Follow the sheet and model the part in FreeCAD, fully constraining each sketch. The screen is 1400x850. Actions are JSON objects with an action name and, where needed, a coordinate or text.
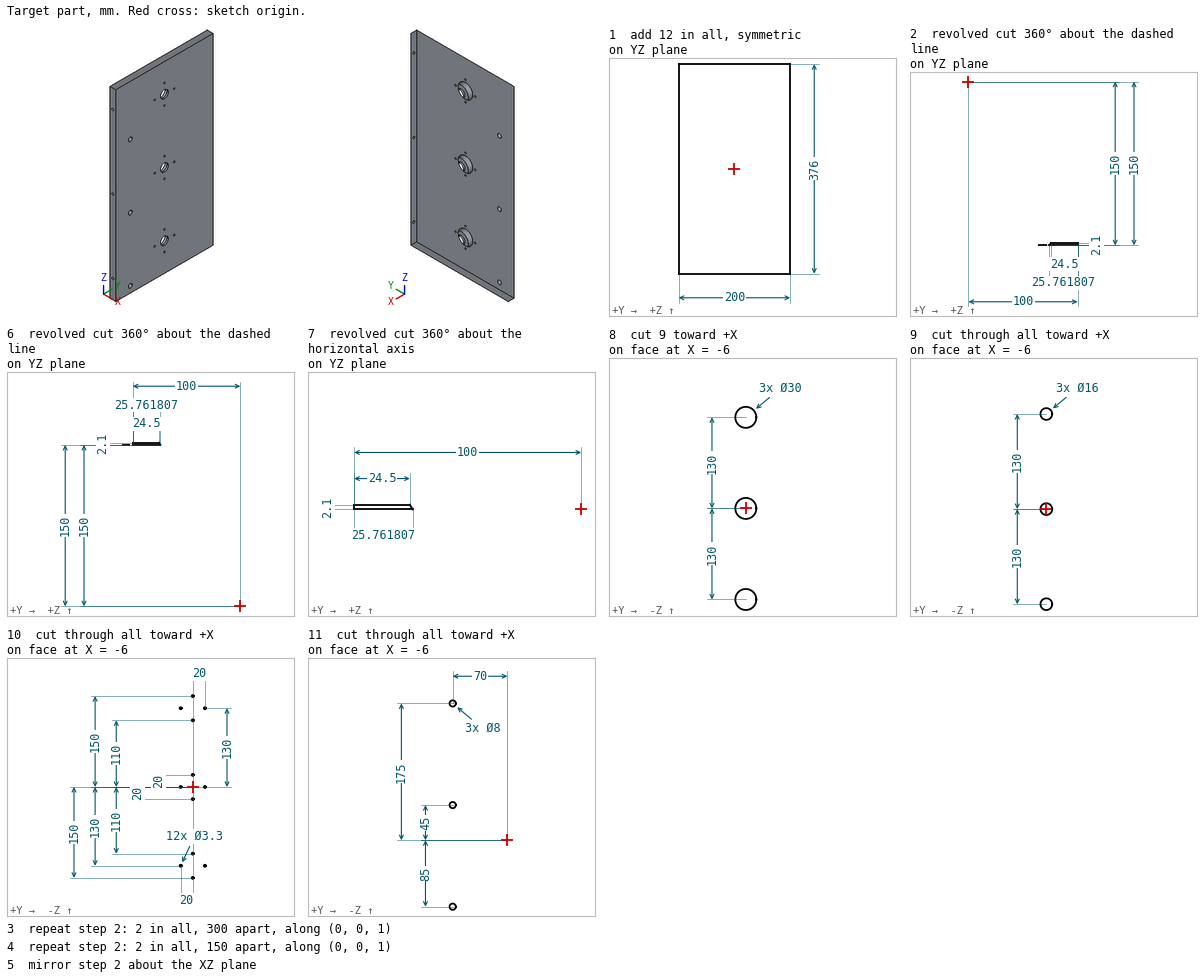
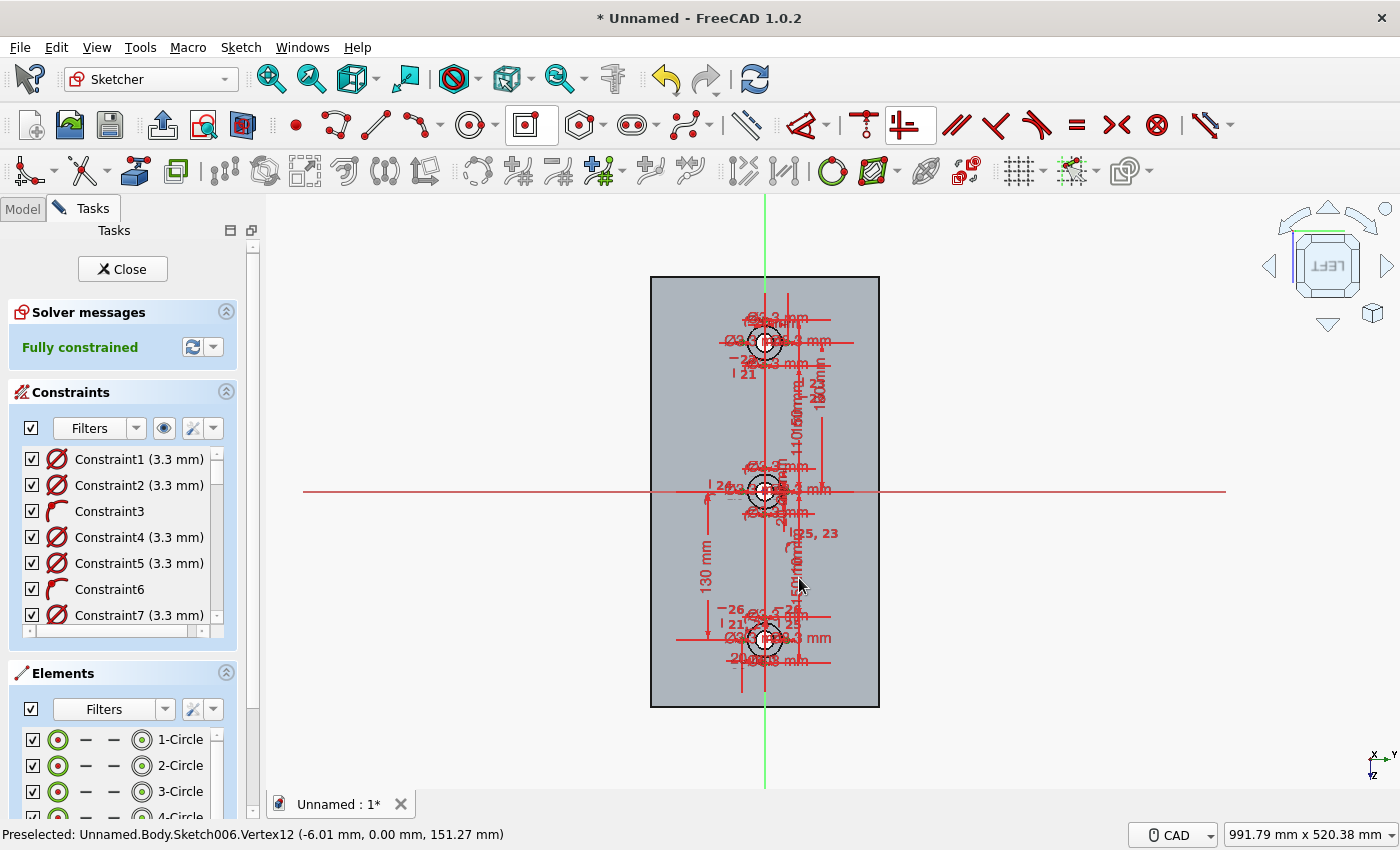
{"action": "left_click", "coordinate": [123, 269]}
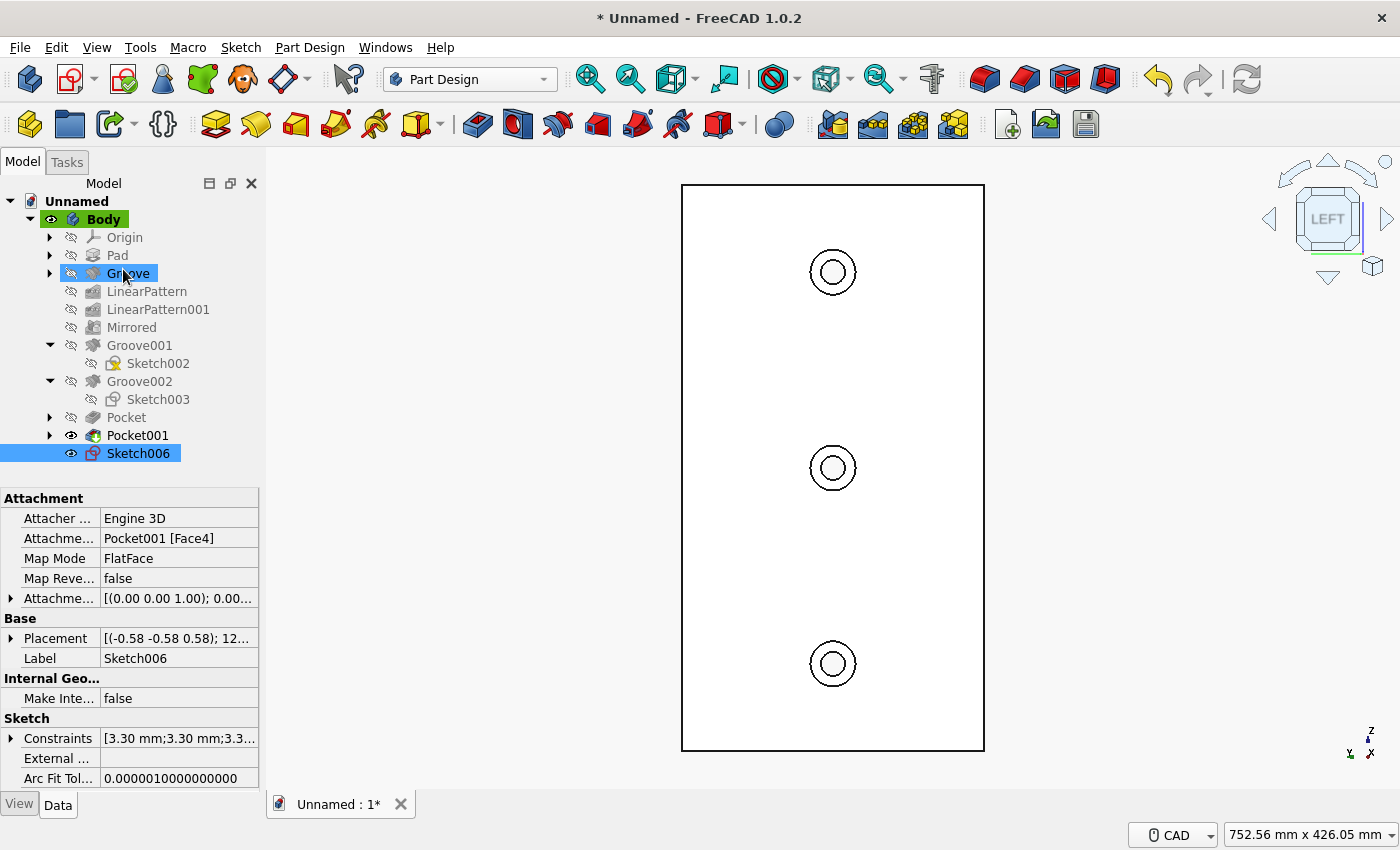
{"action": "left_click", "coordinate": [478, 124]}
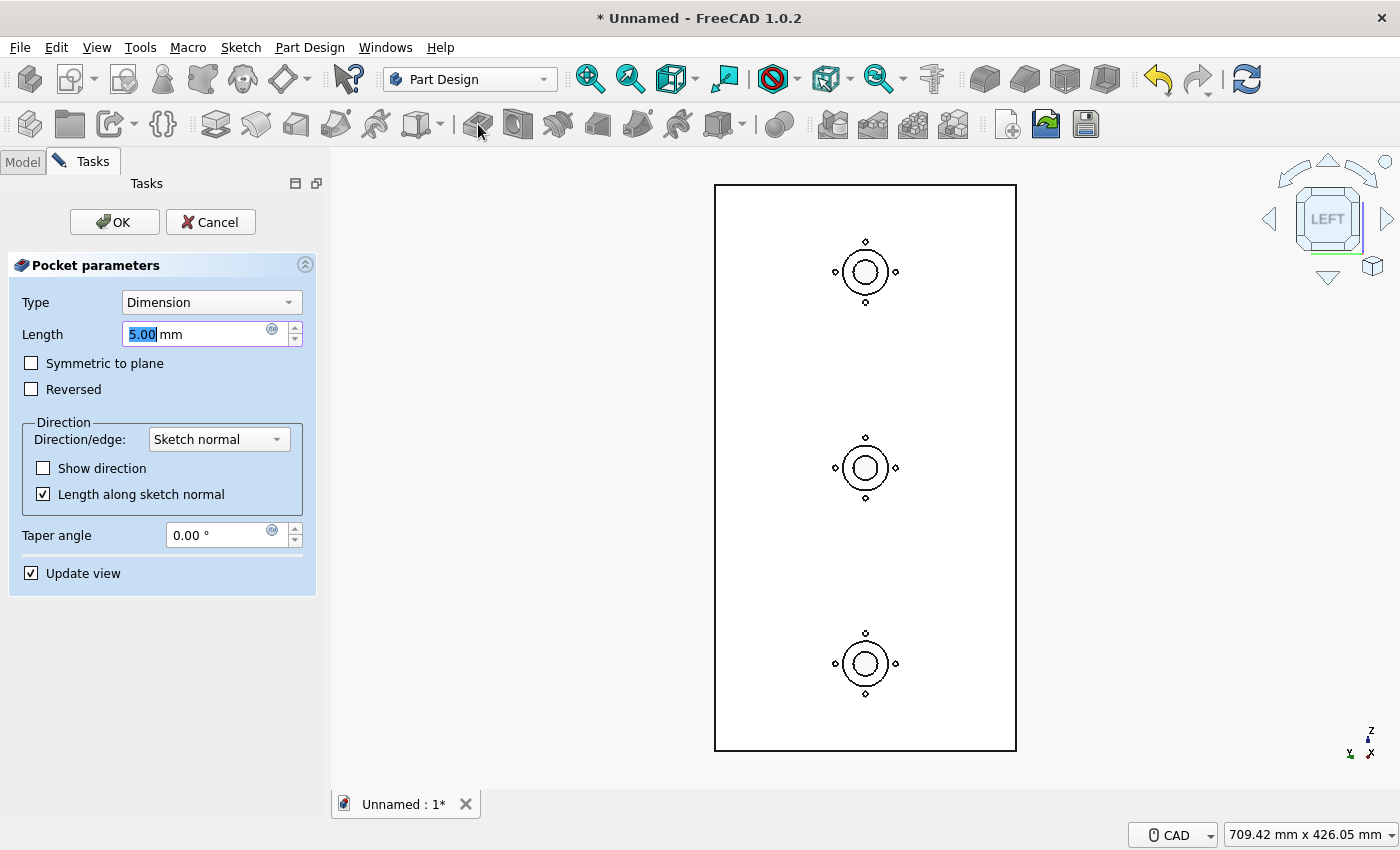
{"action": "left_click", "coordinate": [212, 302]}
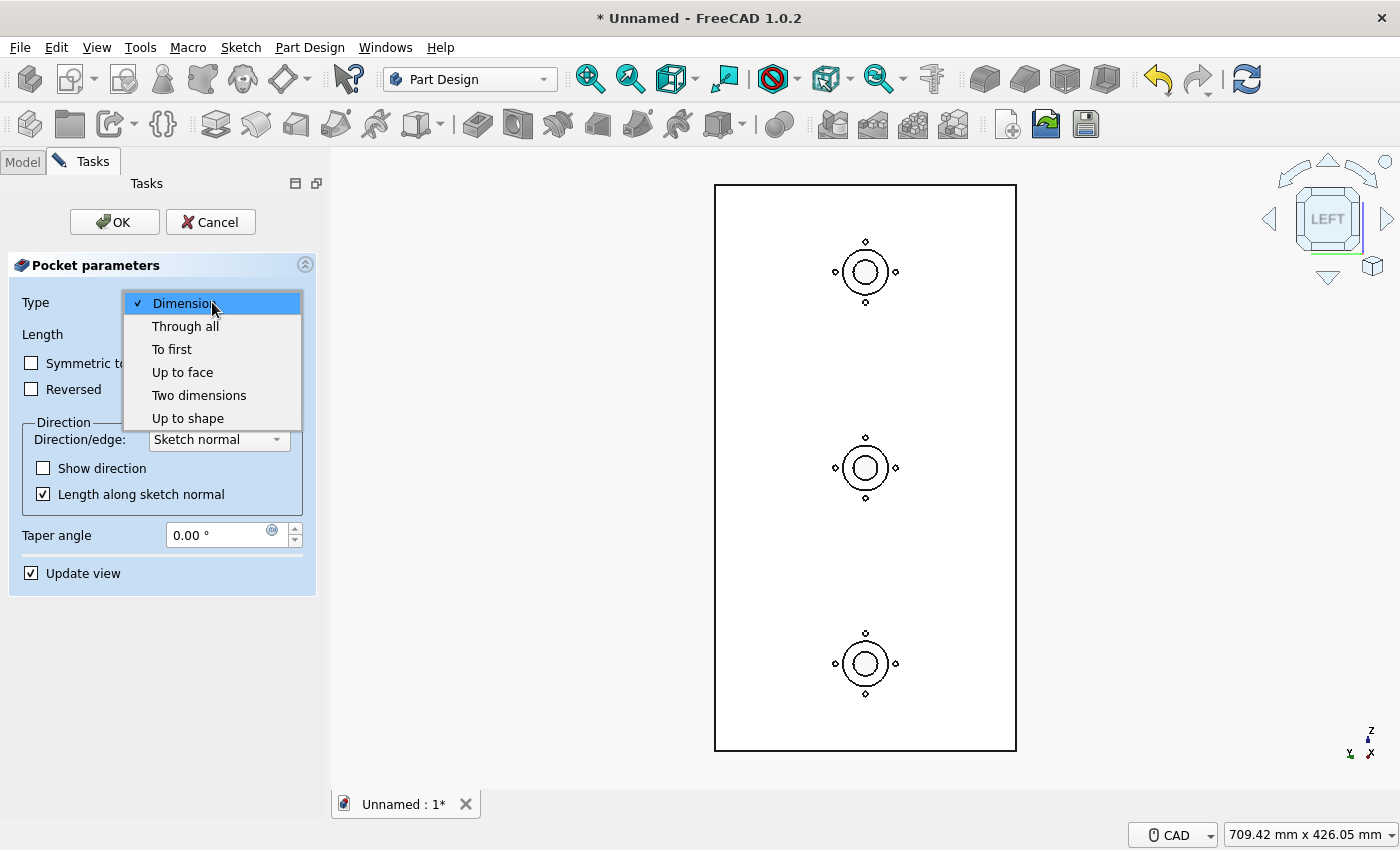
{"action": "left_click", "coordinate": [212, 326]}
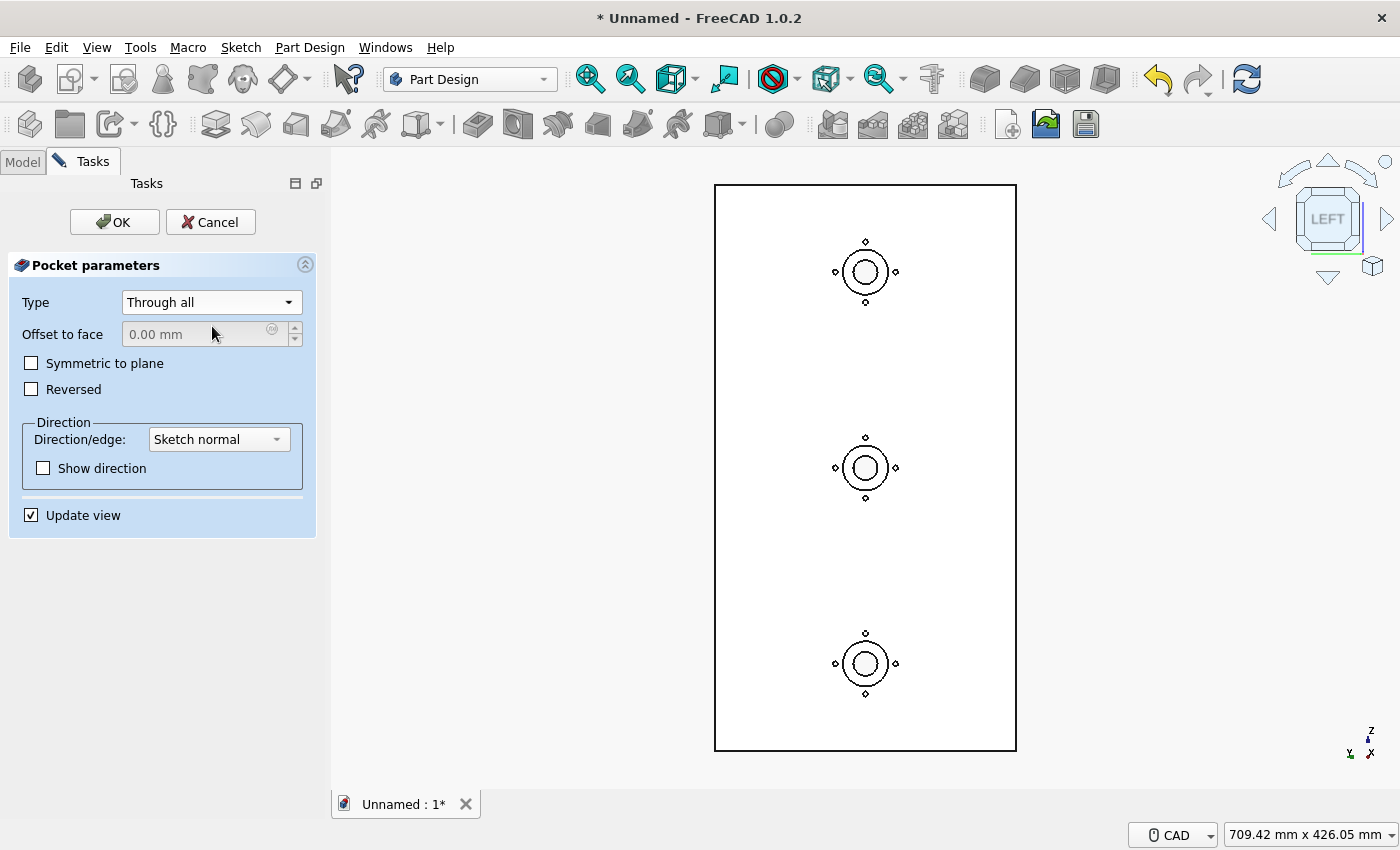
{"action": "left_click", "coordinate": [115, 222]}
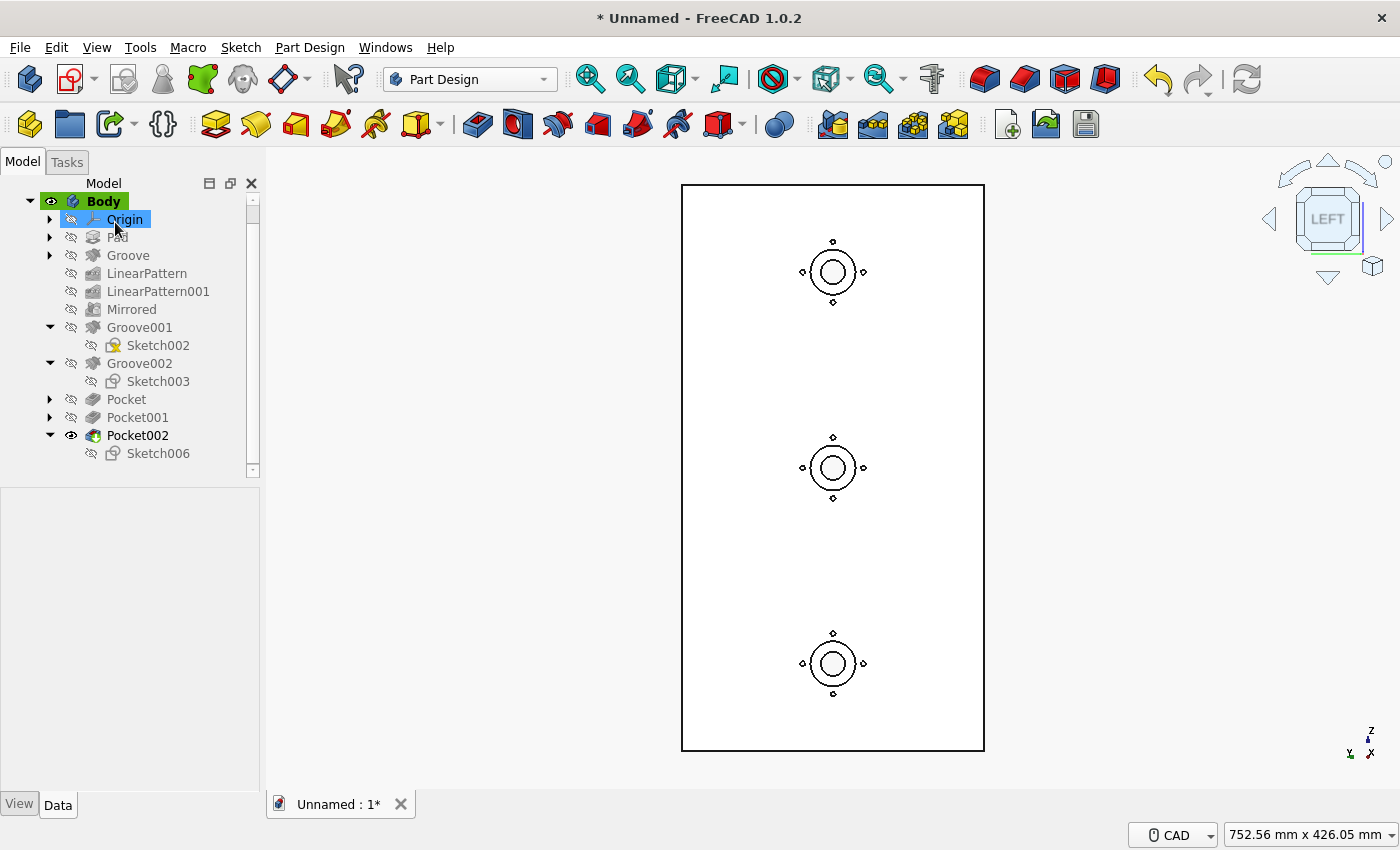
{"action": "left_click", "coordinate": [747, 548]}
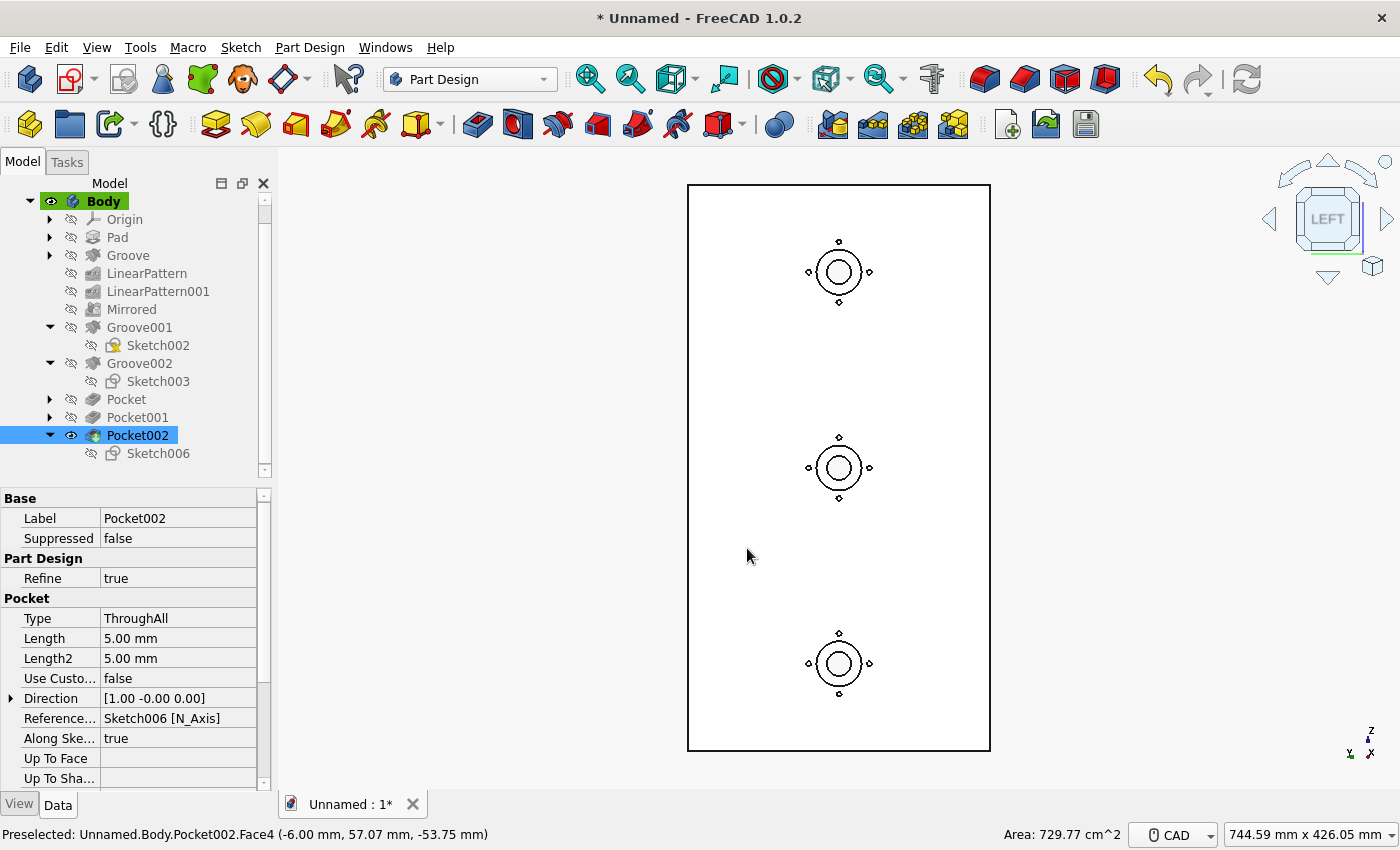
{"action": "left_click", "coordinate": [70, 80]}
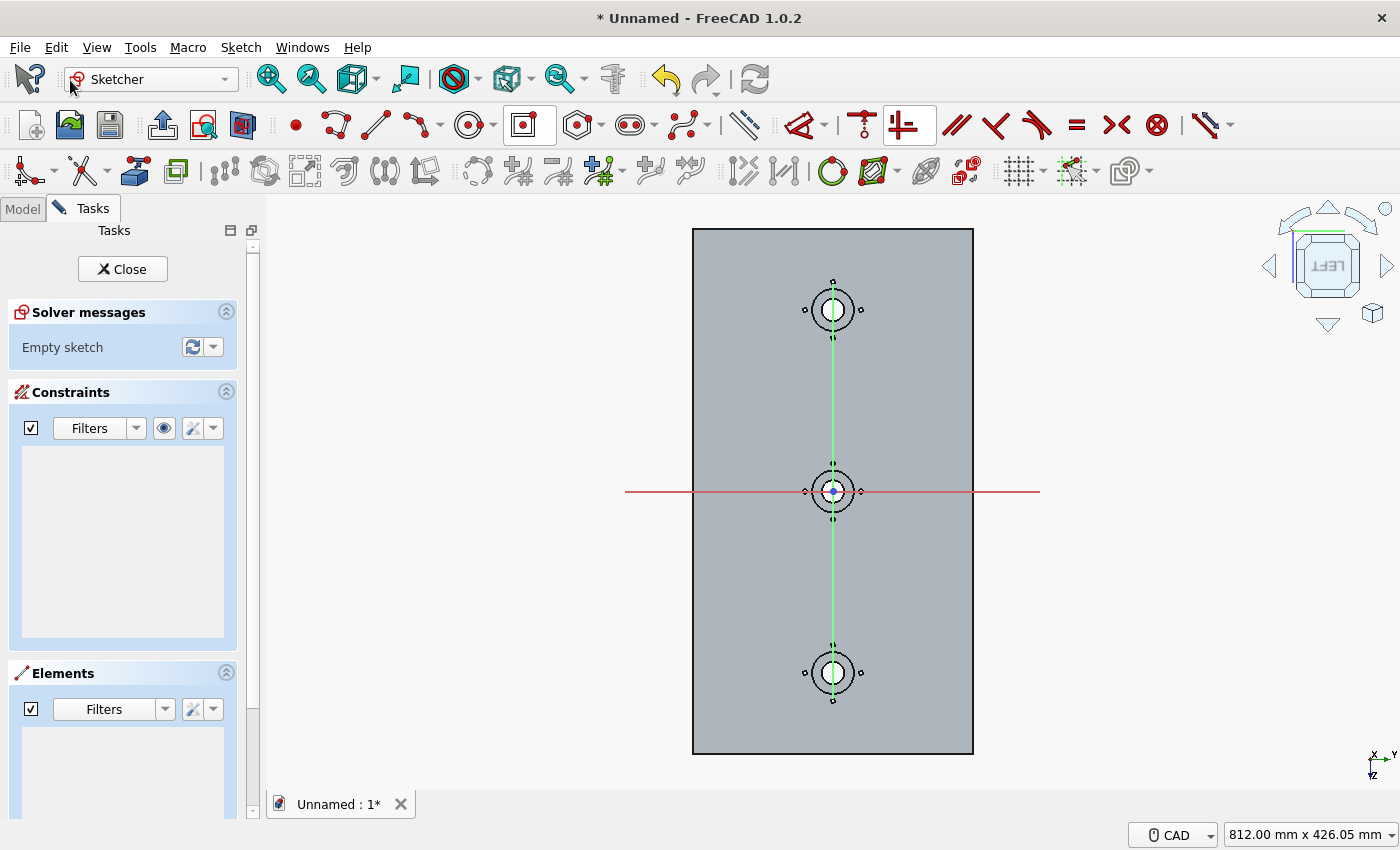
{"action": "scroll", "coordinate": [688, 761], "scroll_direction": "down", "scroll_amount": 1}